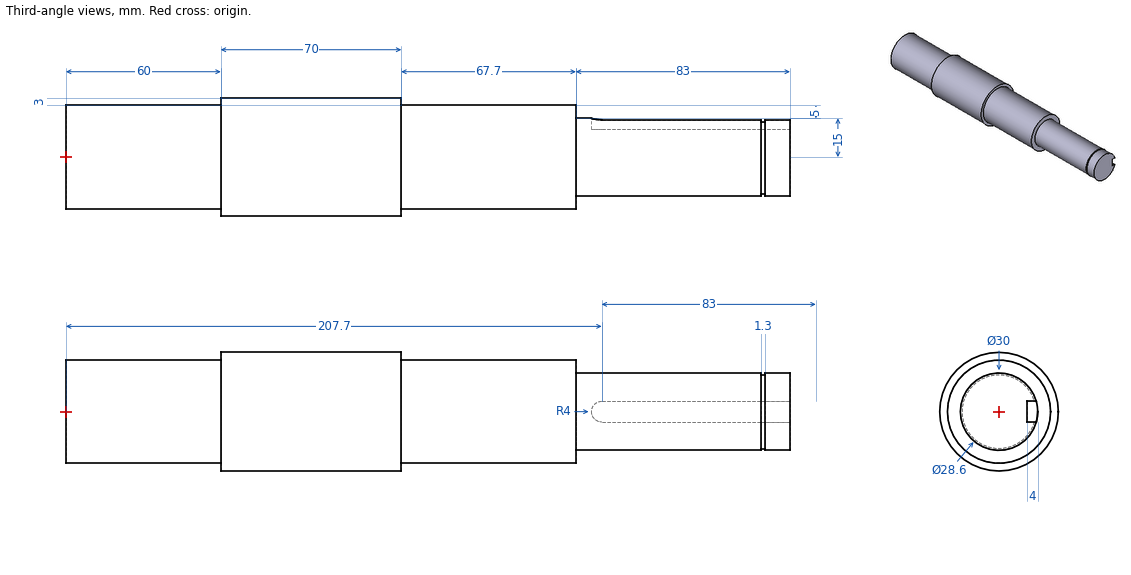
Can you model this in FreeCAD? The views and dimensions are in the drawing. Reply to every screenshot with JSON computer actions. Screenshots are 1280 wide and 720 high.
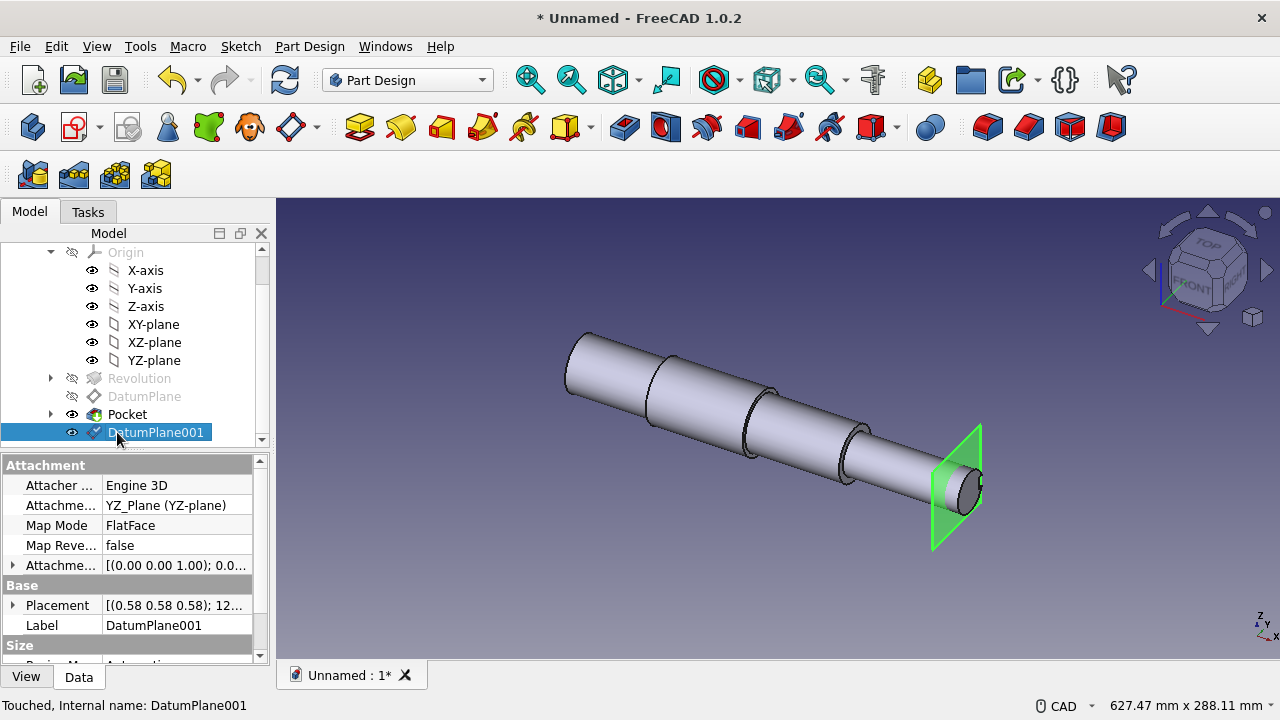
{"action": "left_click", "coordinate": [74, 128]}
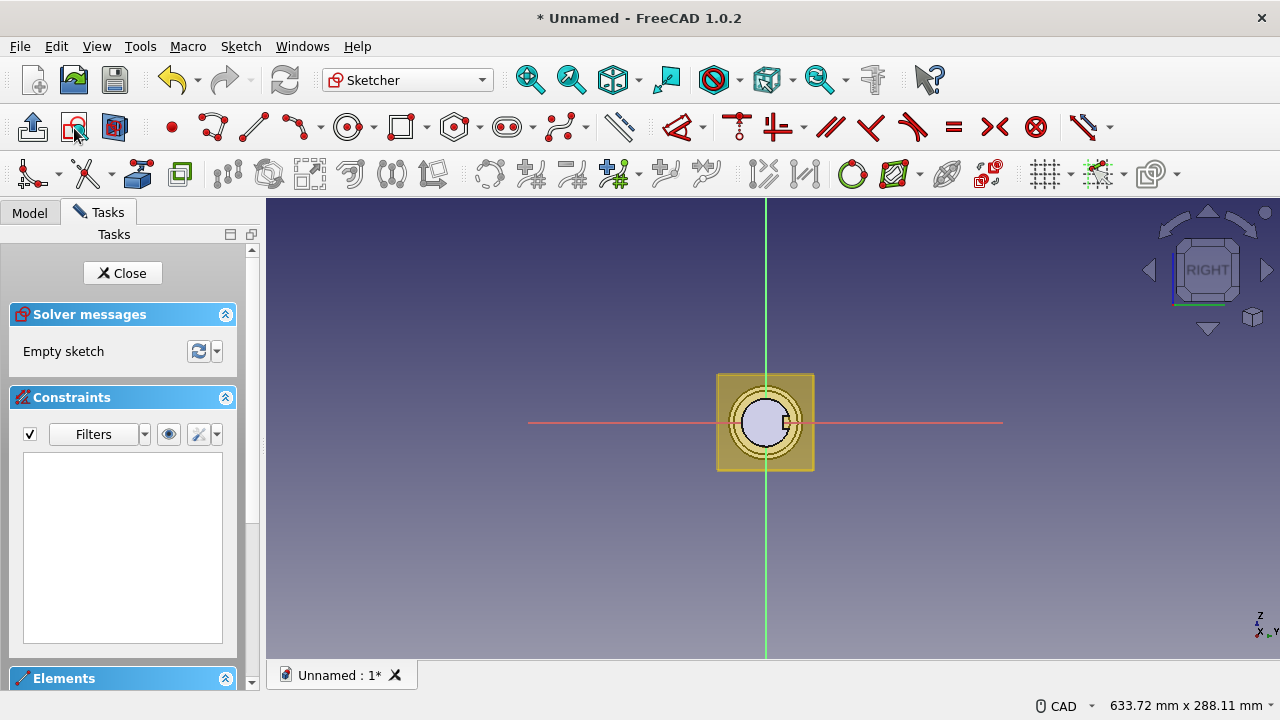
{"action": "key", "text": "q s"}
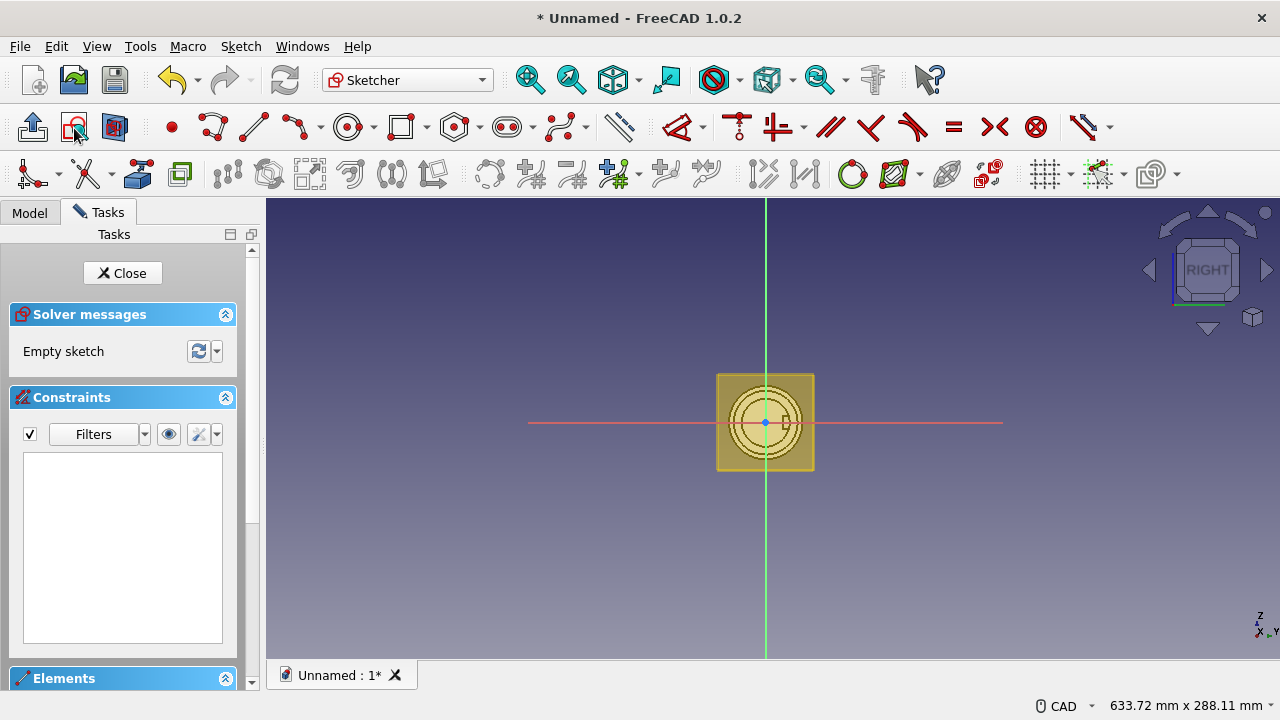
{"action": "scroll", "coordinate": [778, 422], "scroll_direction": "up", "scroll_amount": 9}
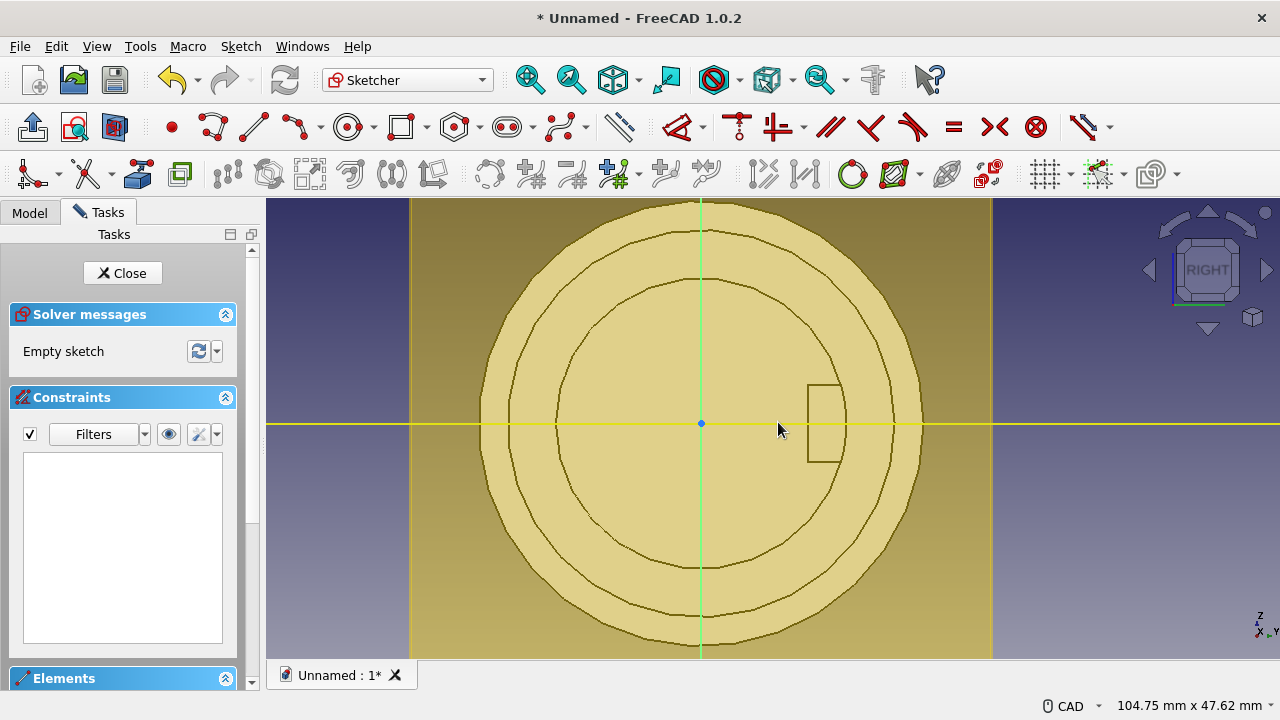
{"action": "key", "text": "g c"}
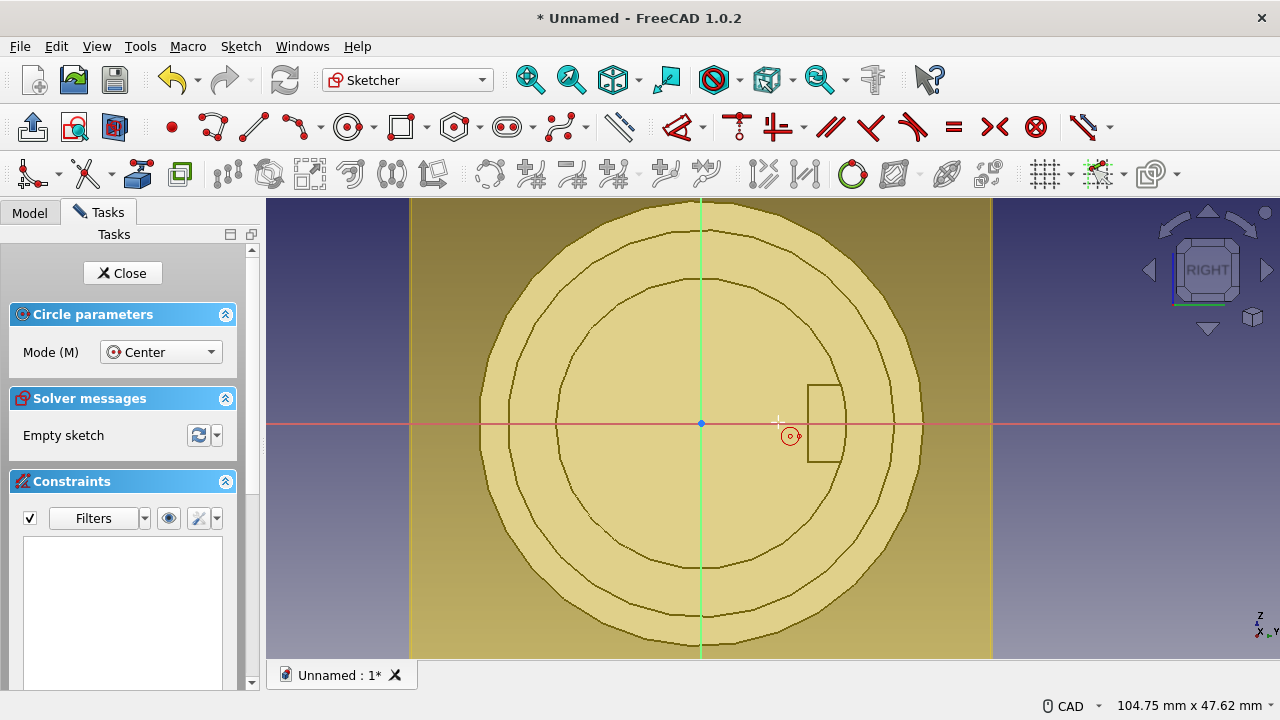
{"action": "left_click", "coordinate": [701, 424]}
{"action": "mouse_move", "coordinate": [804, 321]}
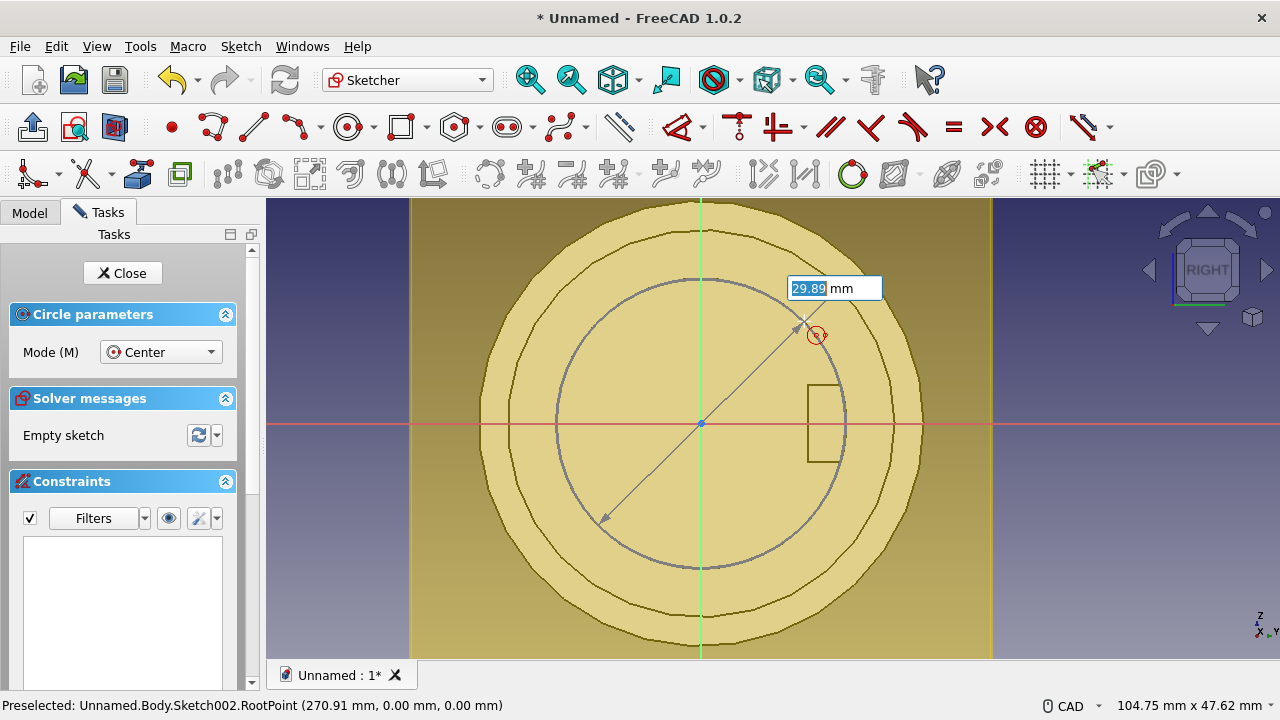
{"action": "type", "text": "30"}
{"action": "key", "text": "Return"}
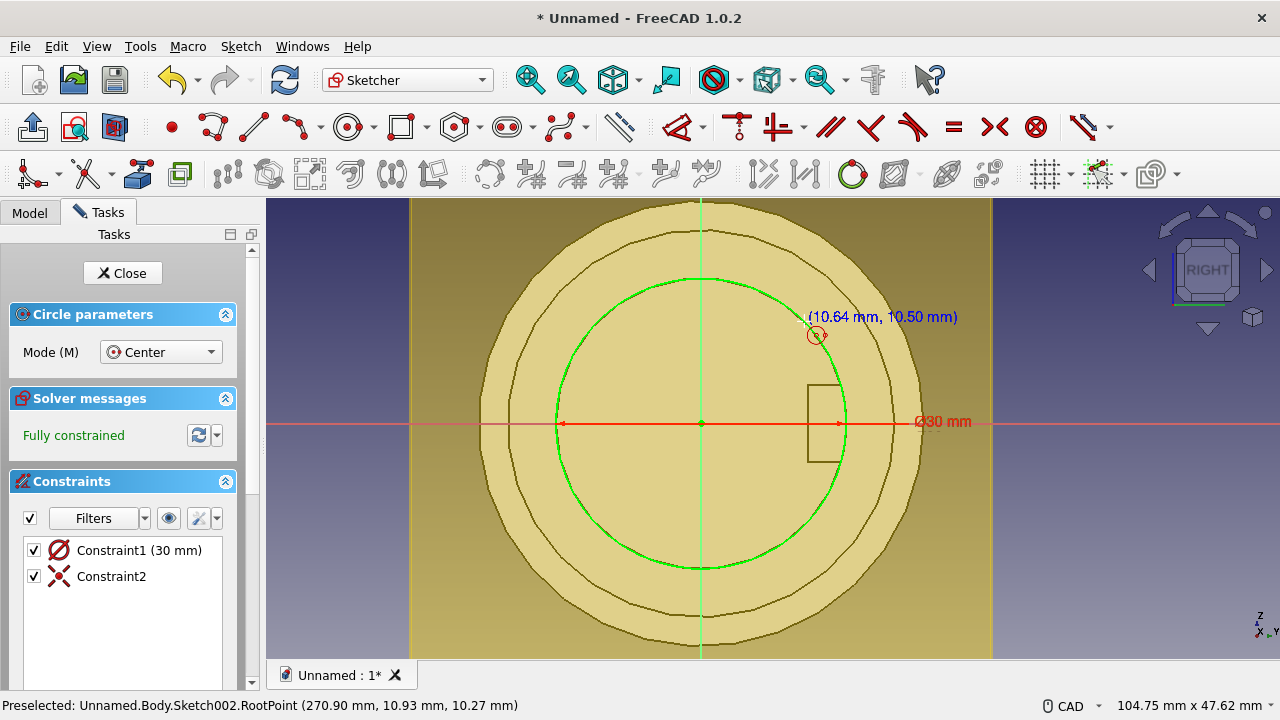
{"action": "left_click", "coordinate": [701, 424]}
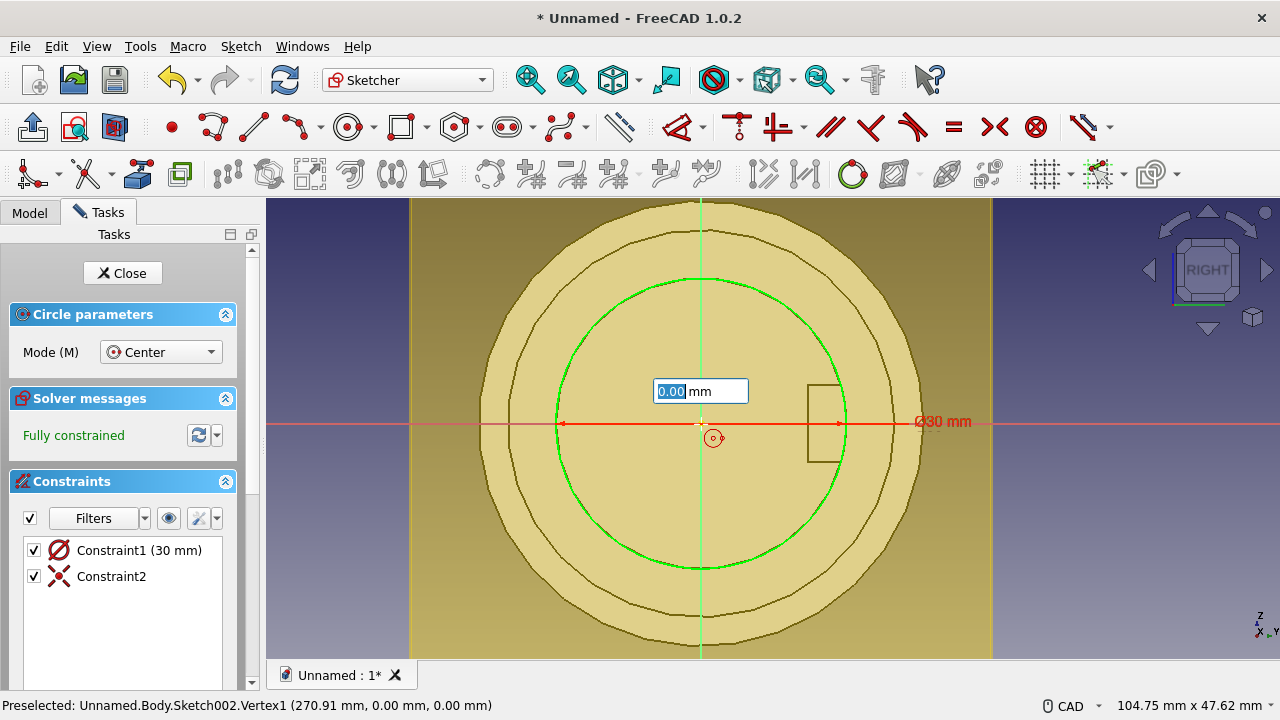
{"action": "scroll", "coordinate": [748, 294], "scroll_direction": "up", "scroll_amount": 5}
{"action": "mouse_move", "coordinate": [748, 292]}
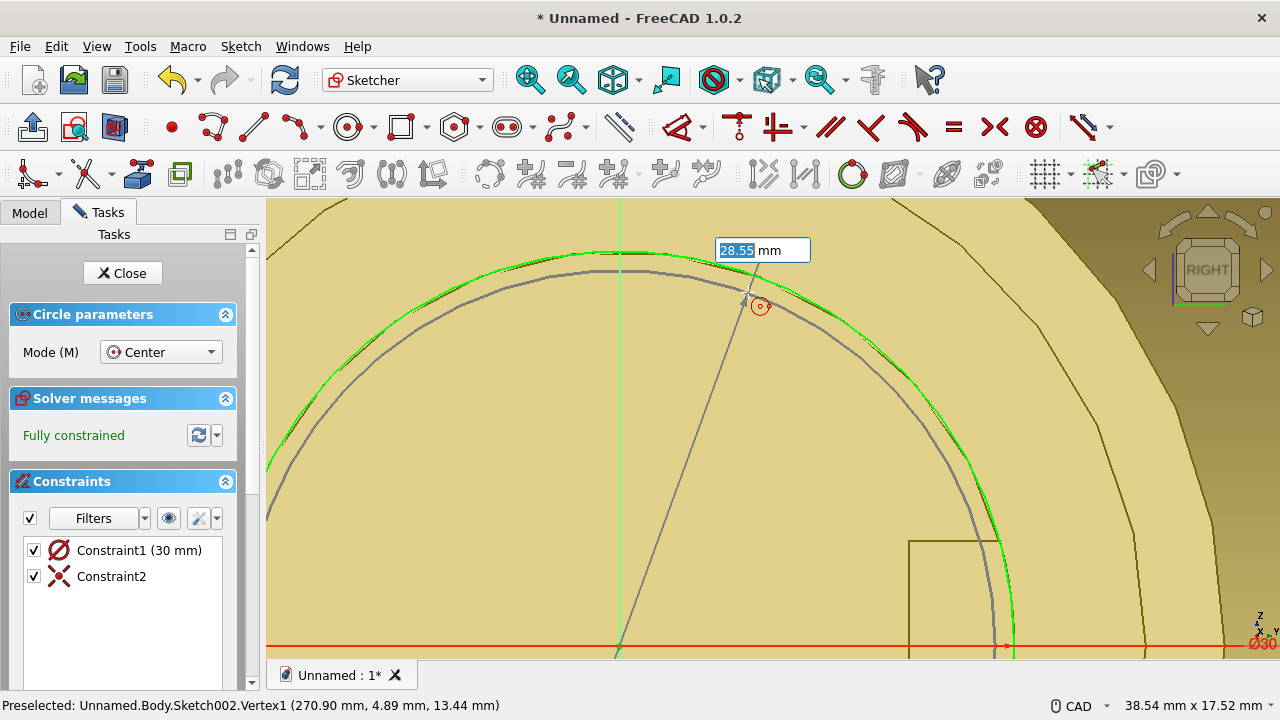
{"action": "type", "text": "28.6"}
{"action": "key", "text": "Return"}
{"action": "key", "text": "Escape"}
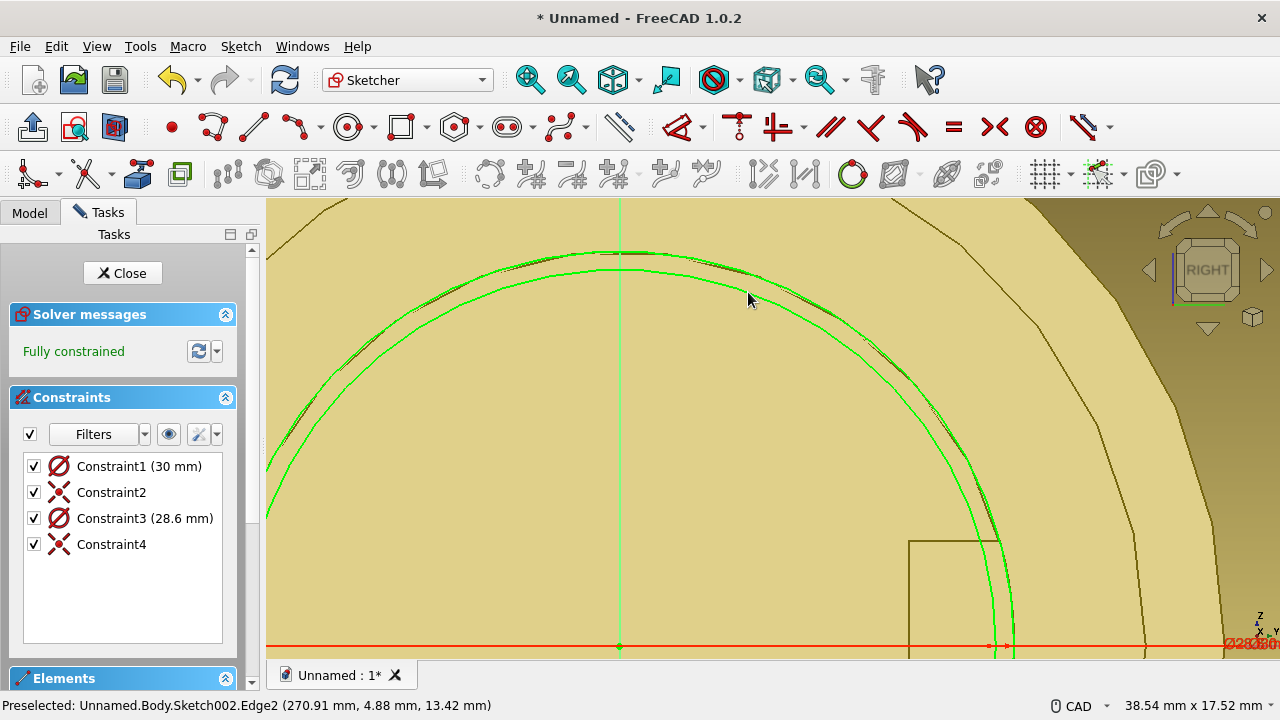
{"action": "left_click", "coordinate": [123, 273]}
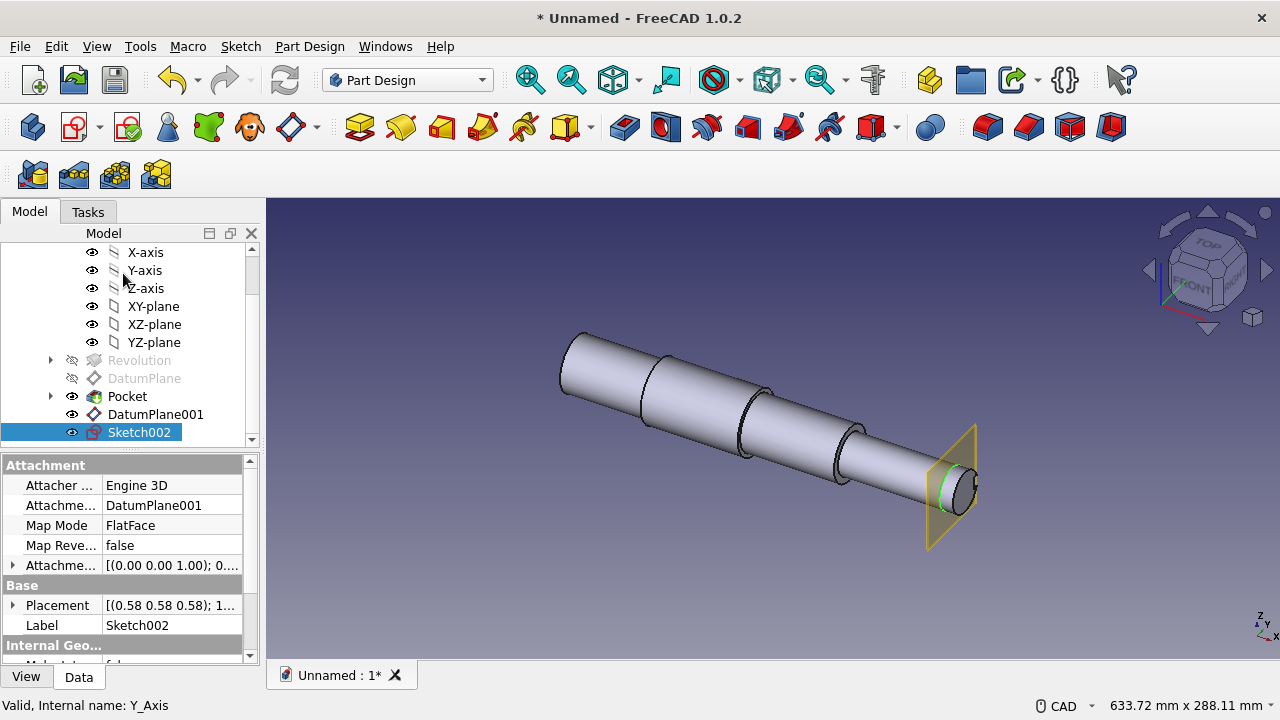
{"action": "left_click", "coordinate": [625, 128]}